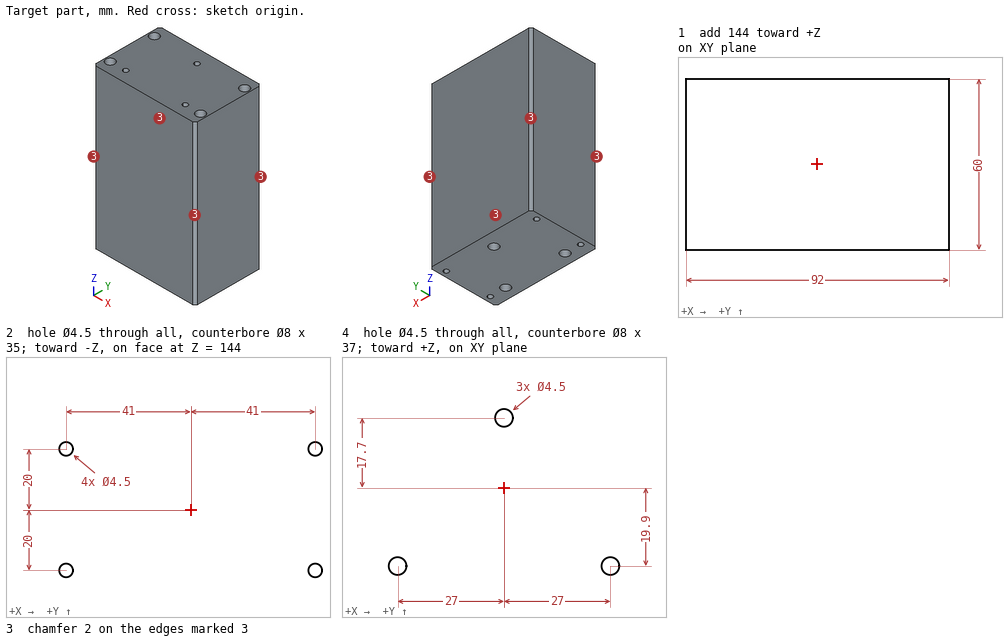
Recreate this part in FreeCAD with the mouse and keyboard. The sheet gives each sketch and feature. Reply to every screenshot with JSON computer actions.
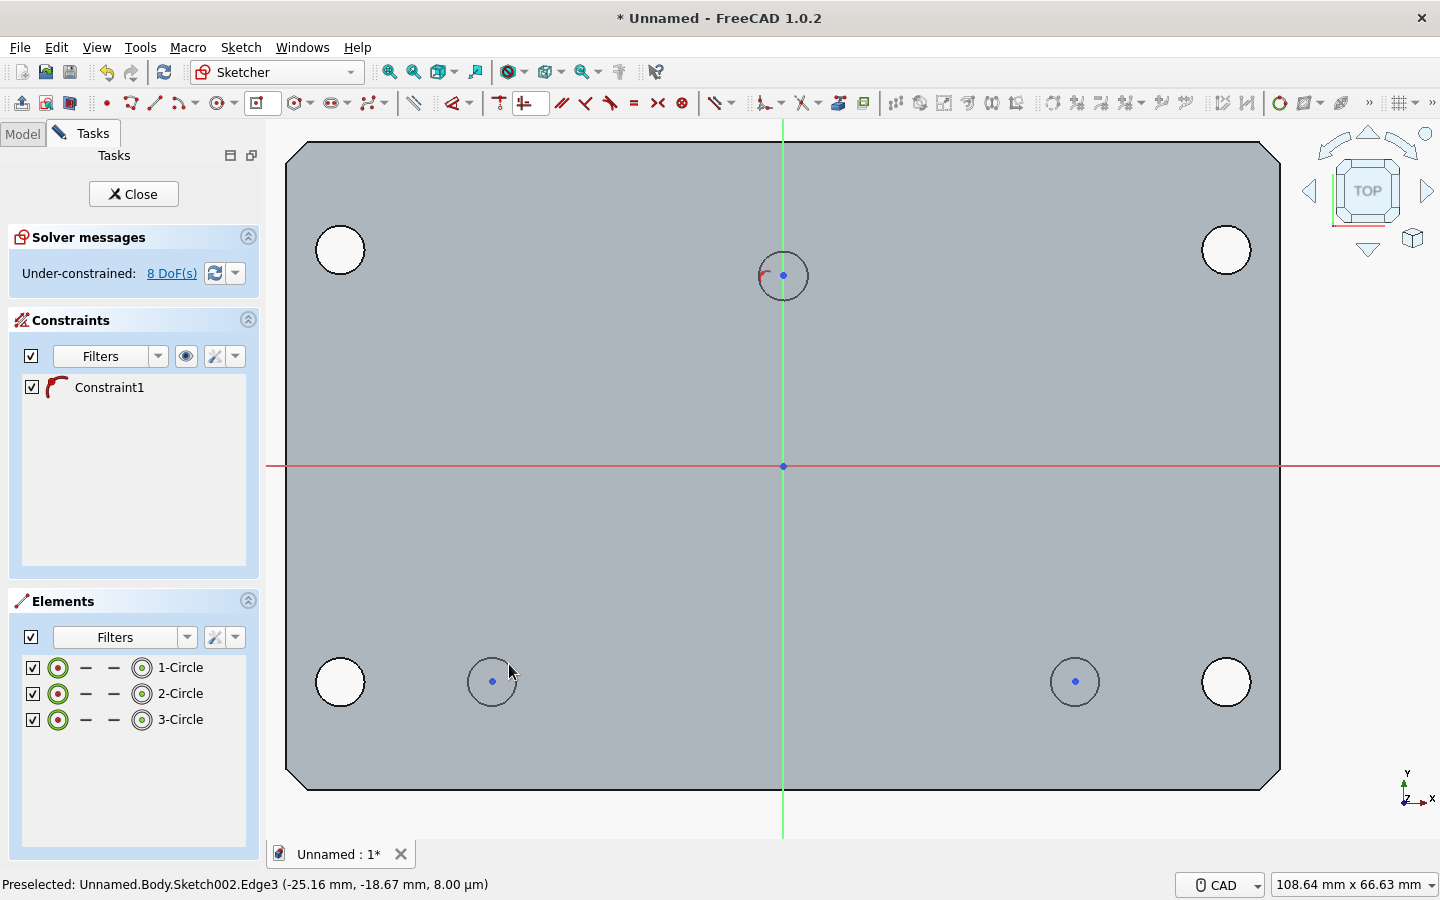
{"action": "left_click", "coordinate": [801, 259]}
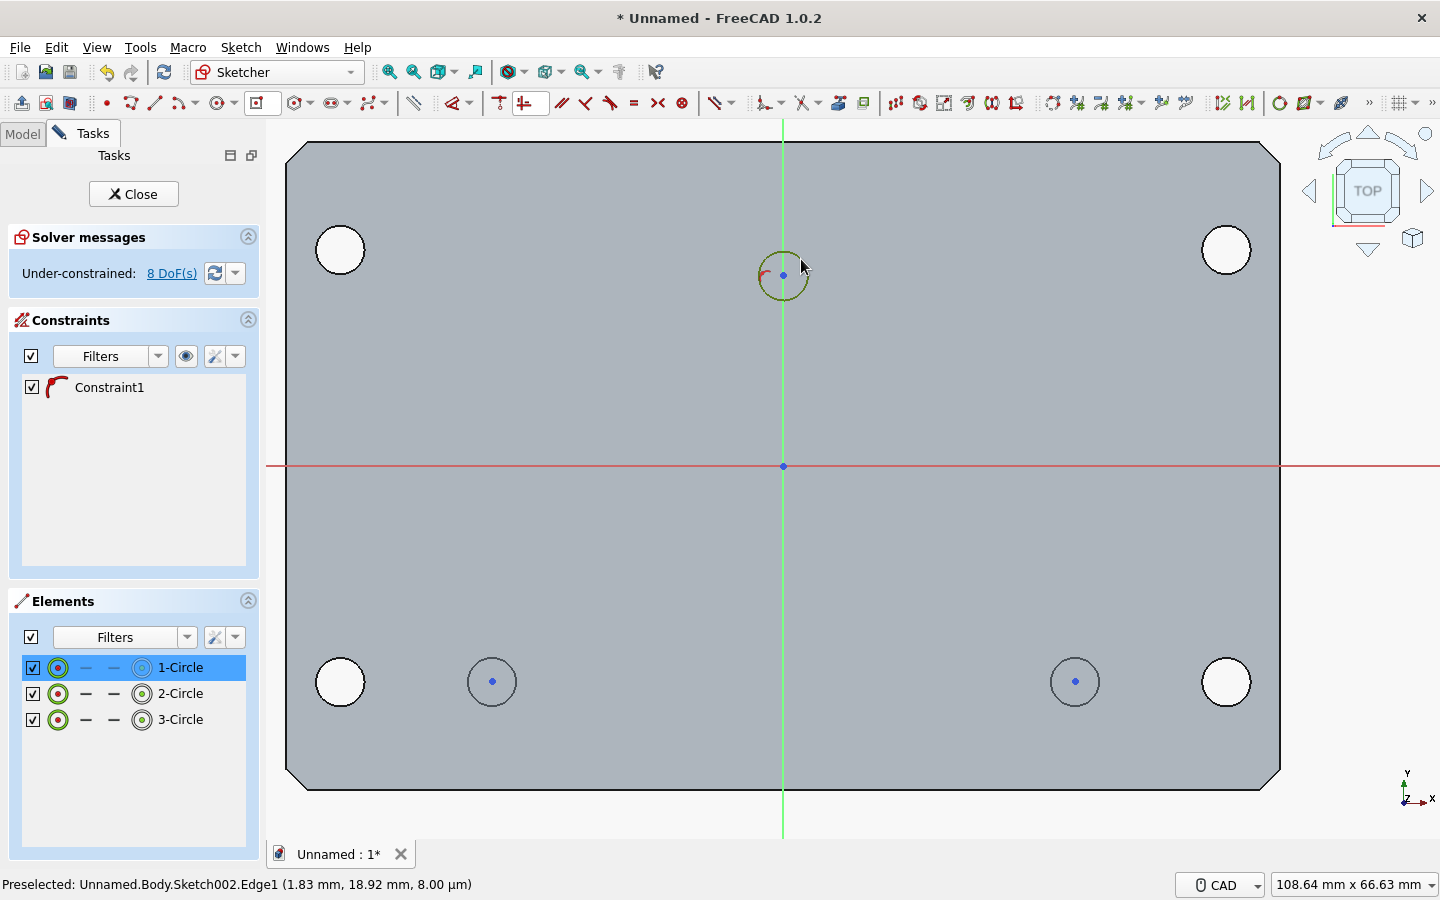
{"action": "left_click", "coordinate": [1092, 665]}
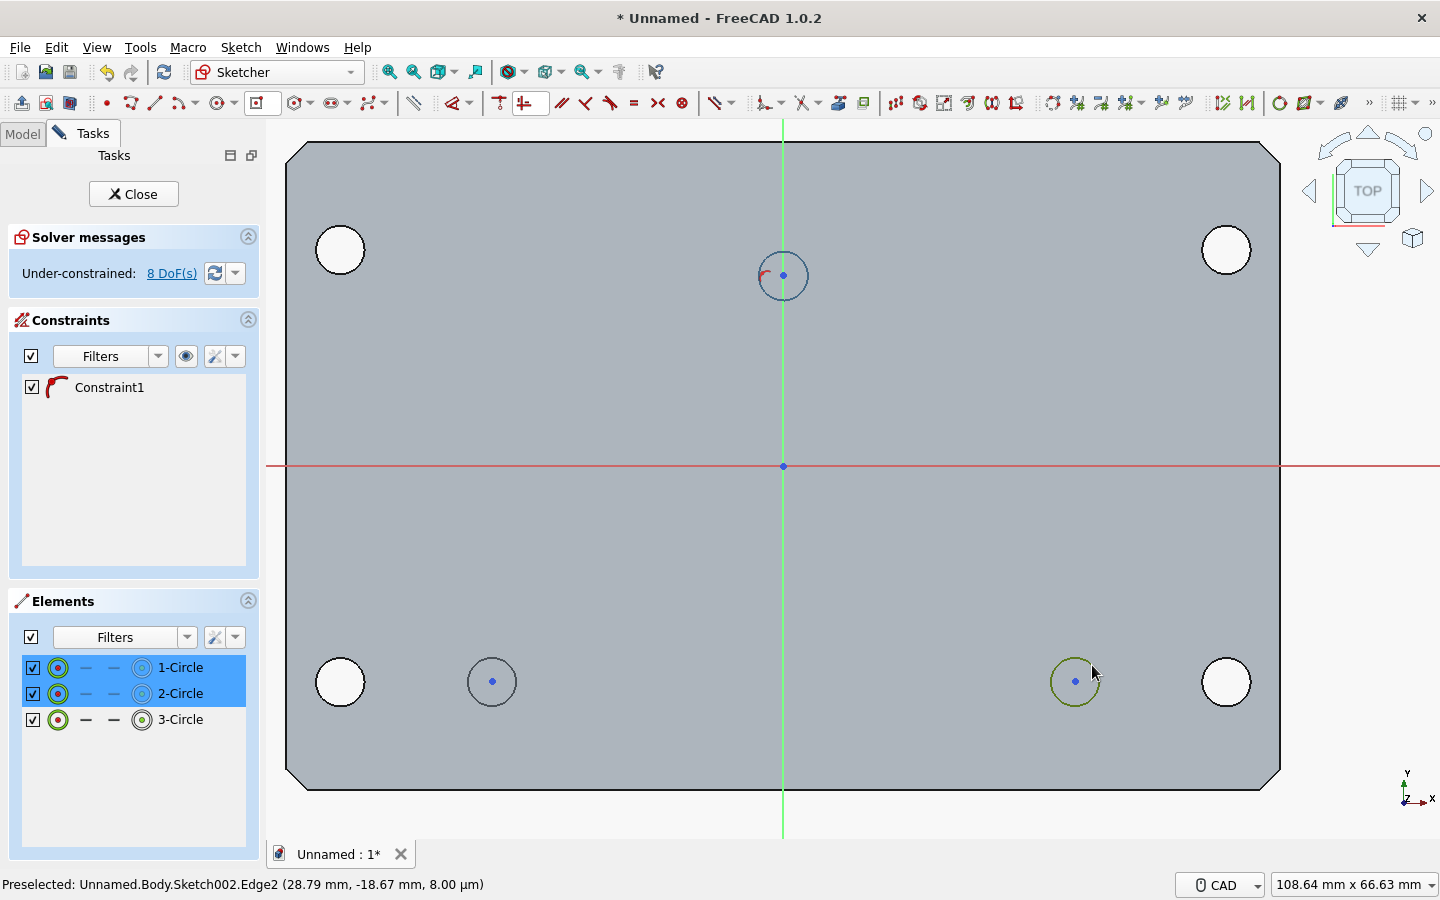
{"action": "left_click", "coordinate": [509, 665]}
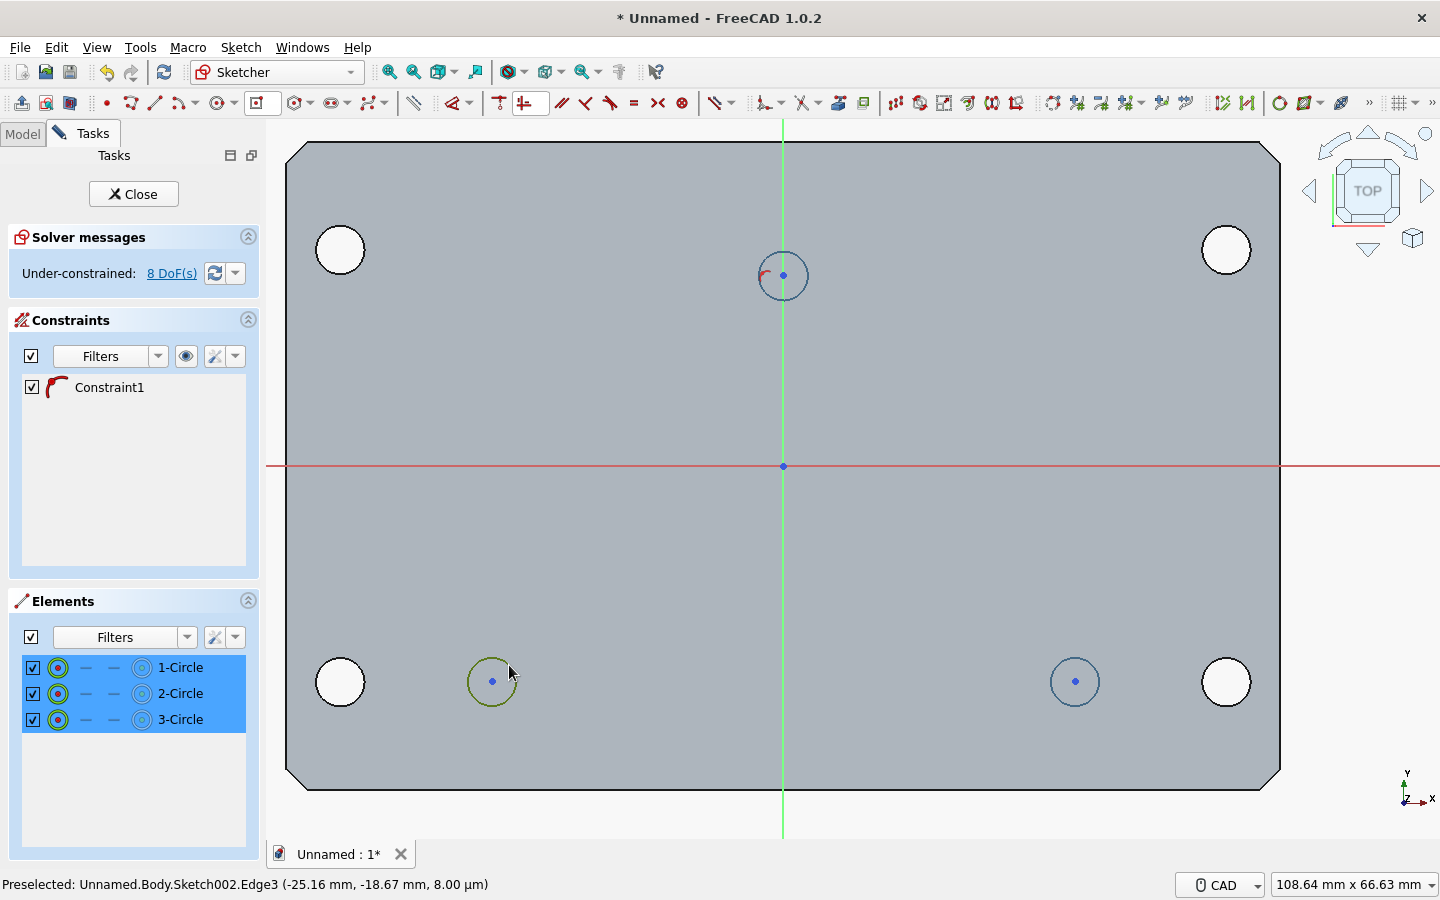
{"action": "left_click", "coordinate": [634, 104]}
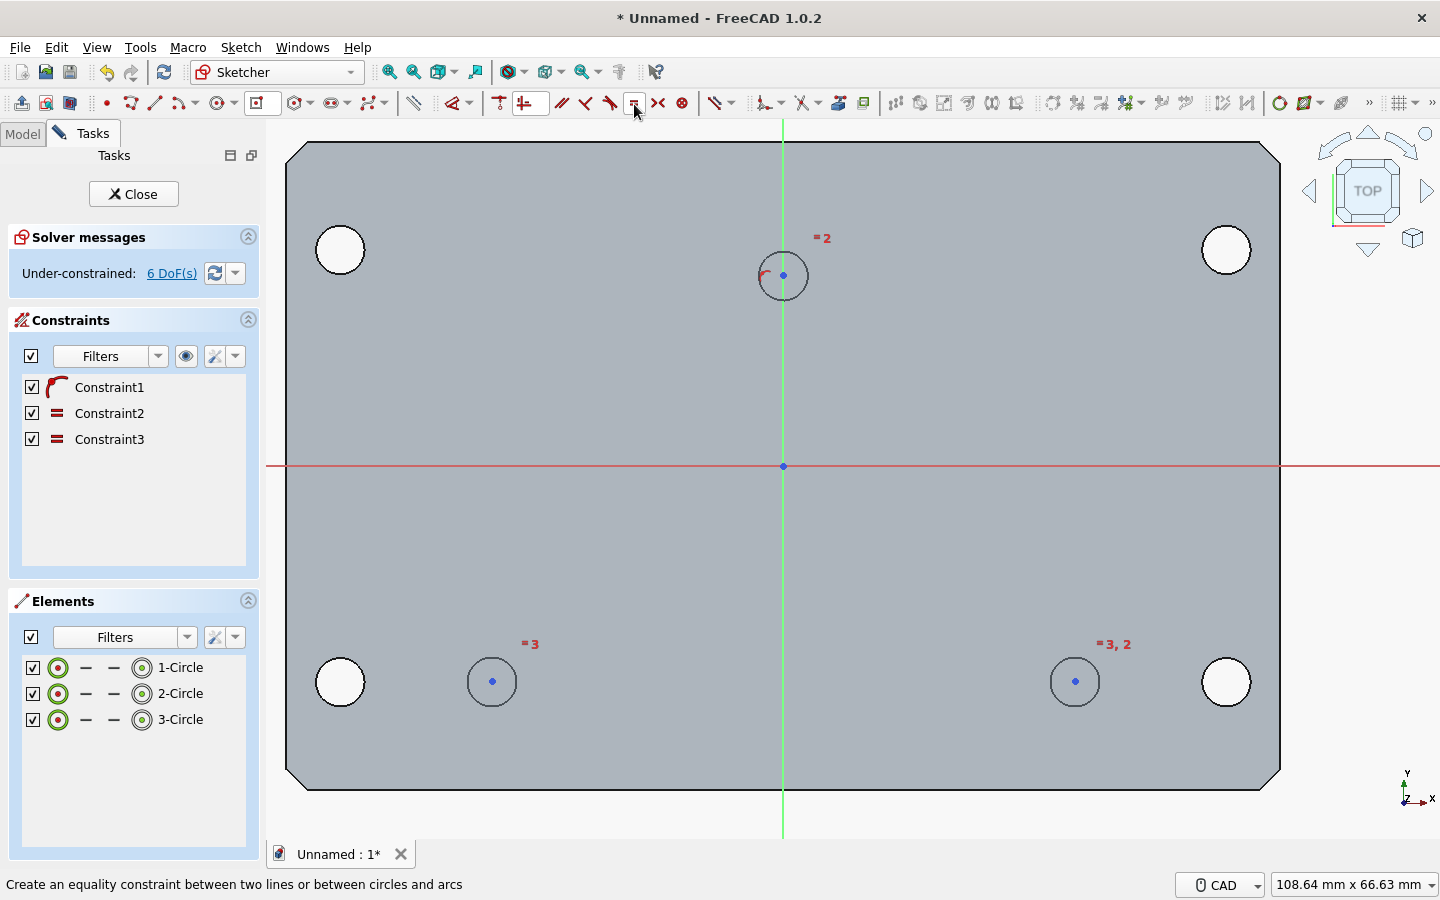
{"action": "left_click", "coordinate": [1075, 682]}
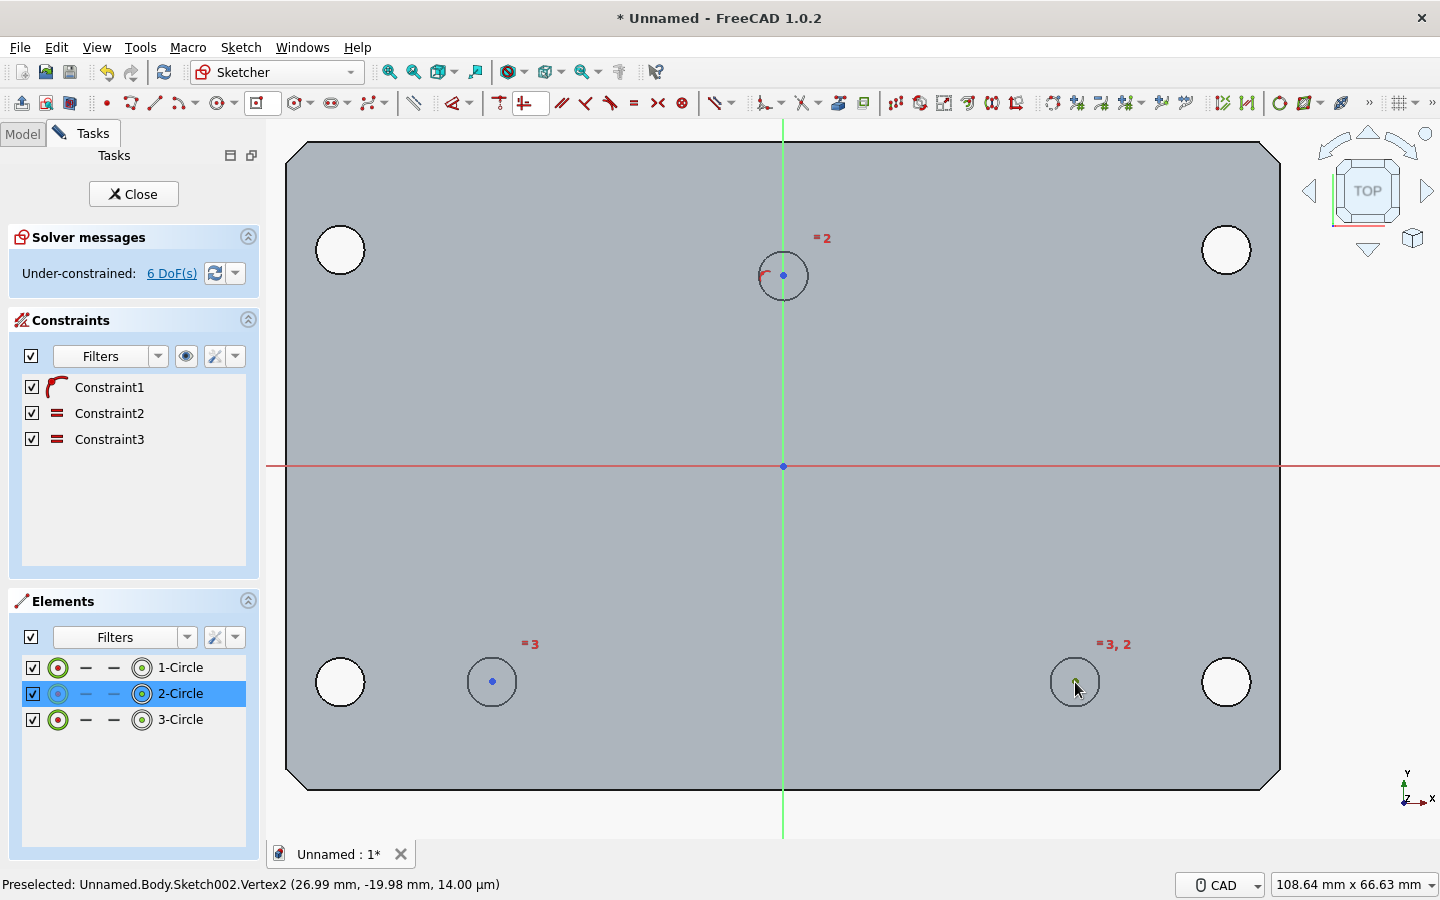
{"action": "left_click", "coordinate": [492, 682]}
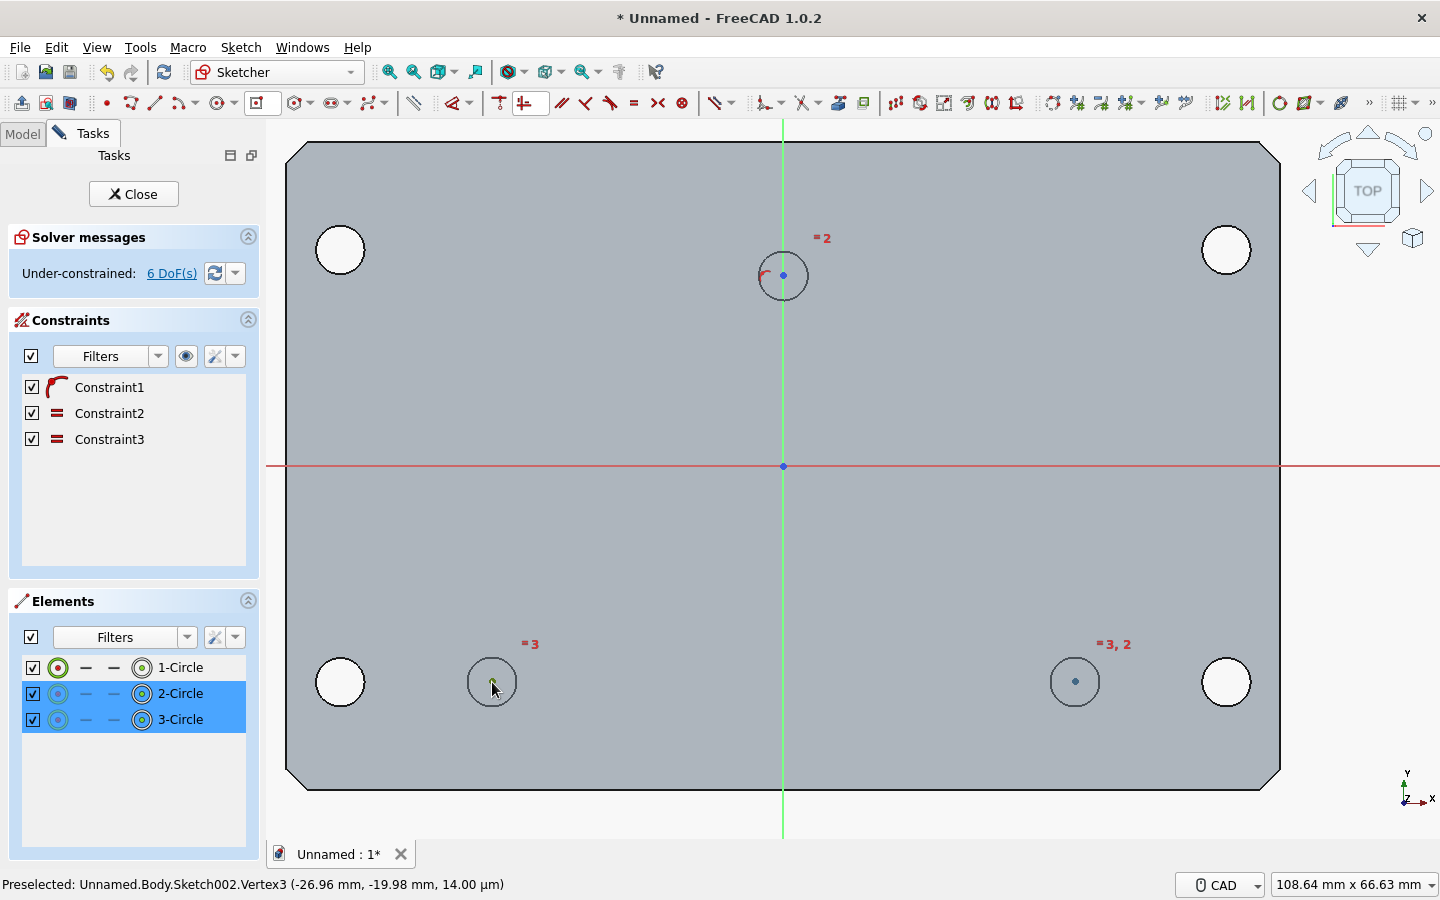
{"action": "key", "text": "h"}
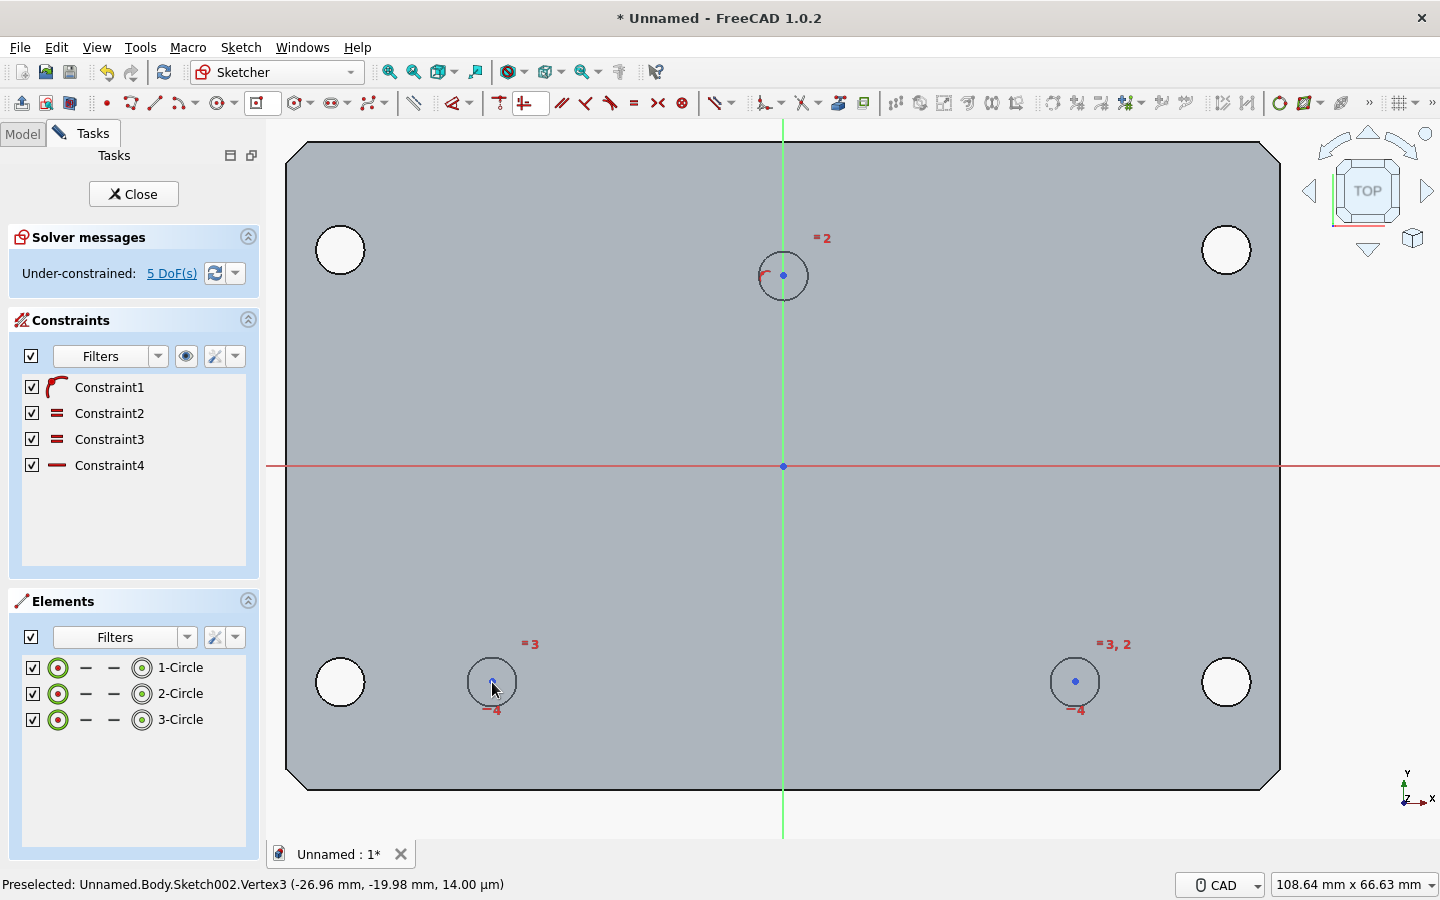
{"action": "left_click", "coordinate": [452, 104]}